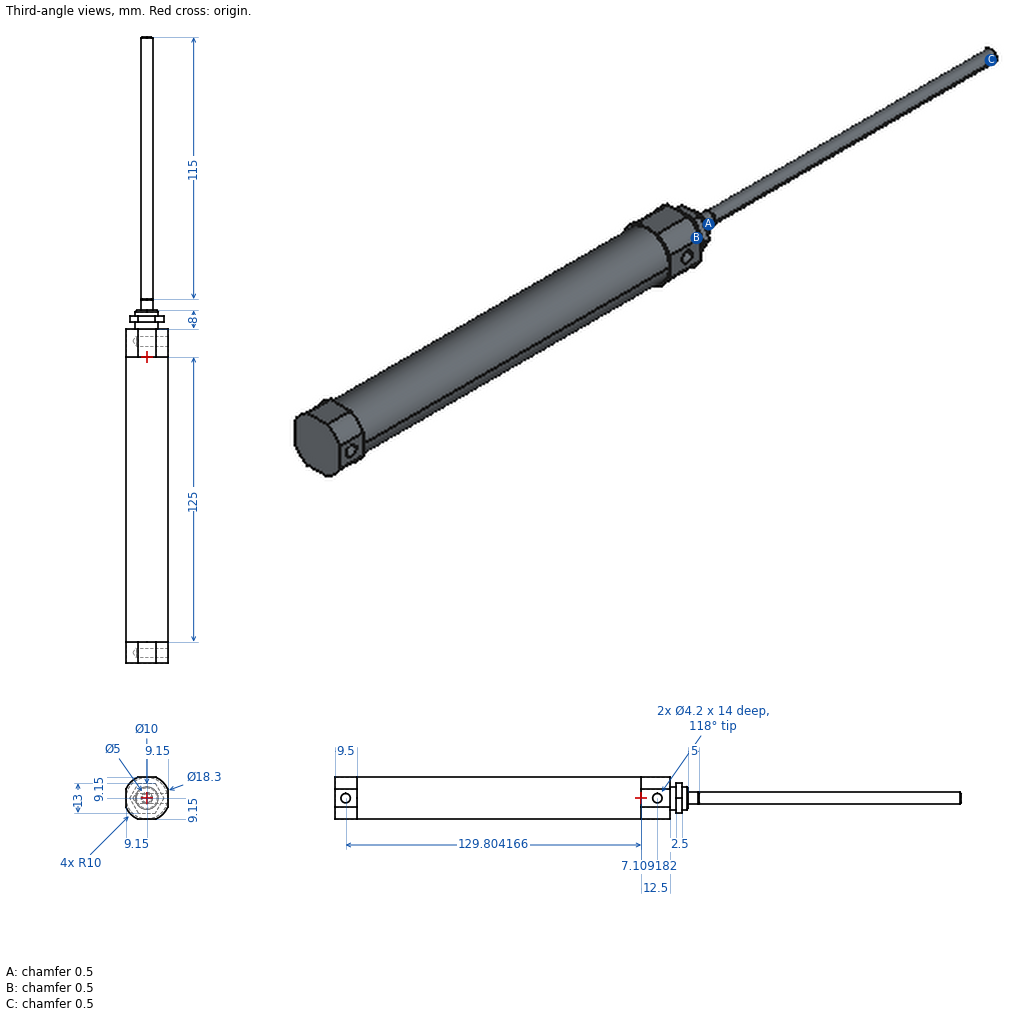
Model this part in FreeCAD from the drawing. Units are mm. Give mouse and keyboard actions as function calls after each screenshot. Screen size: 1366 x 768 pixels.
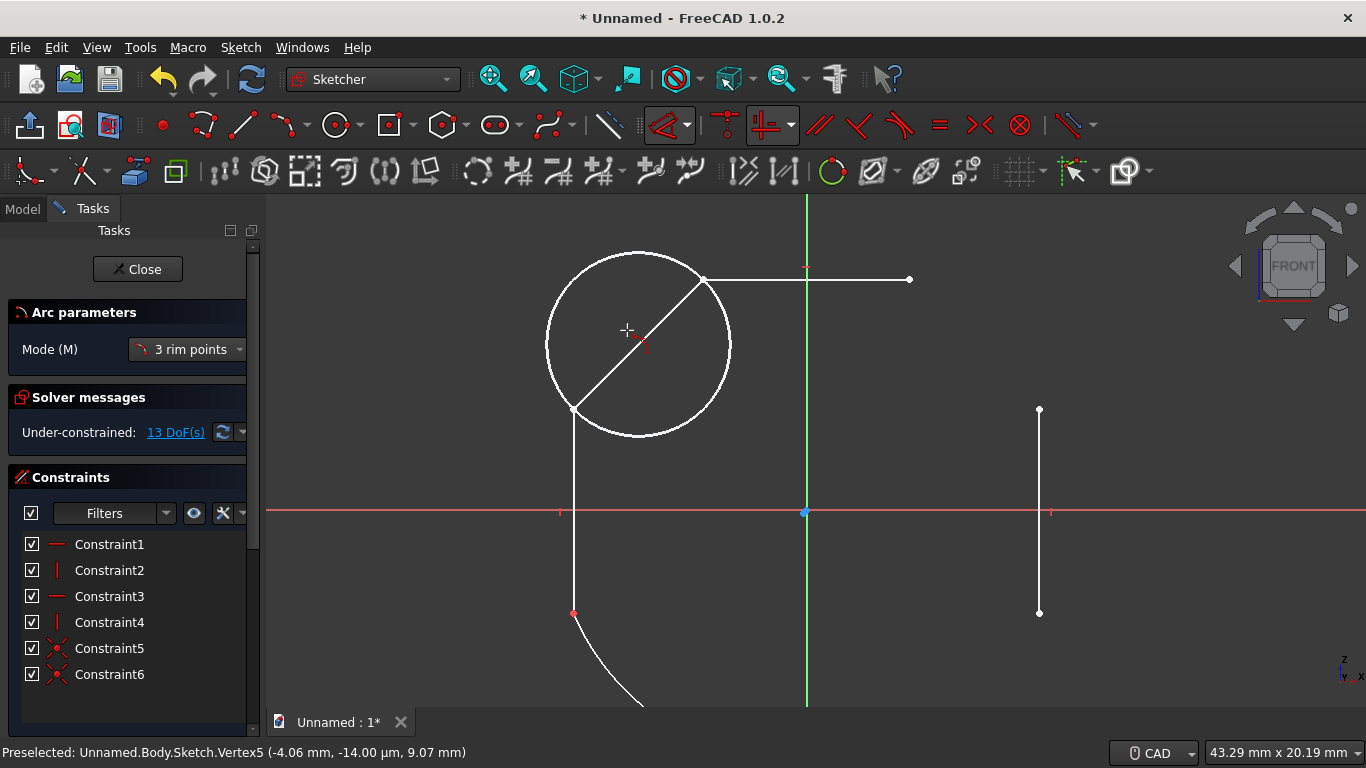
click(627, 330)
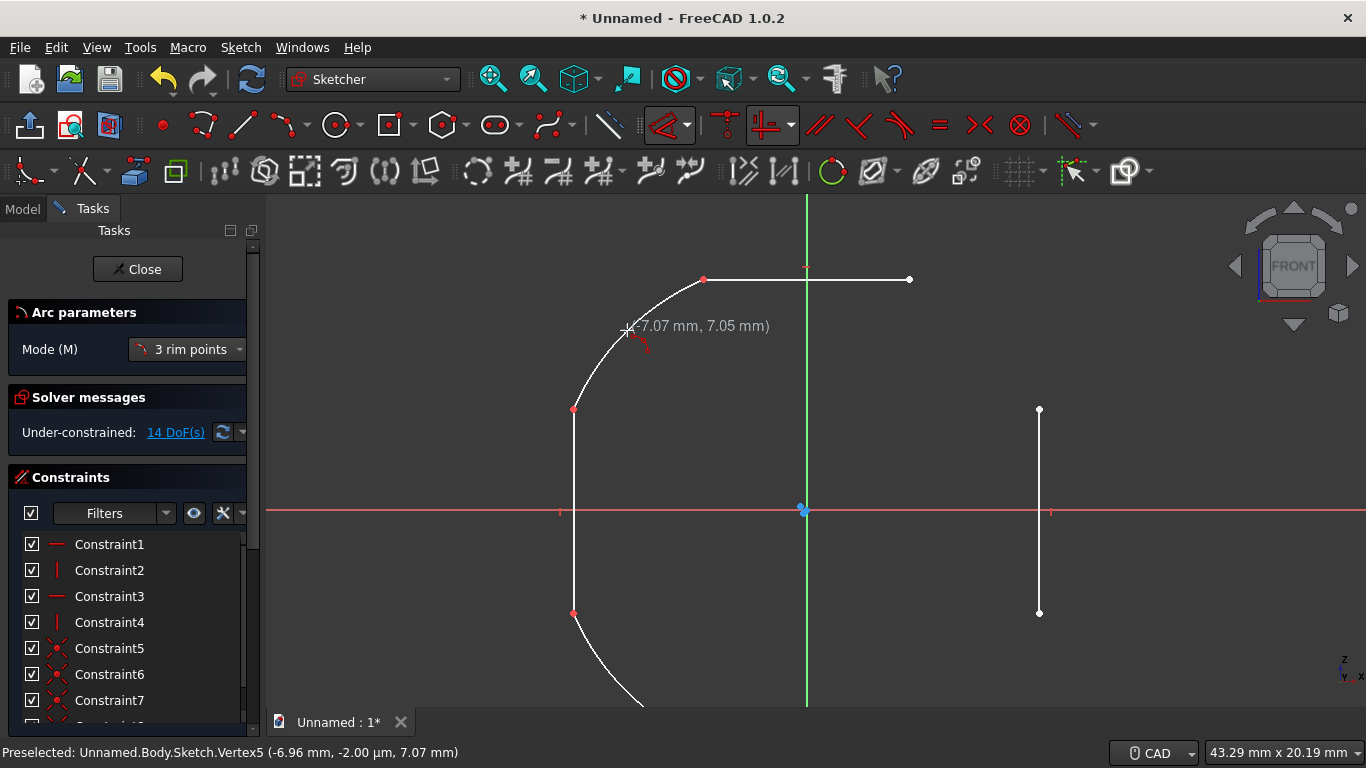
click(909, 280)
click(1039, 409)
click(986, 330)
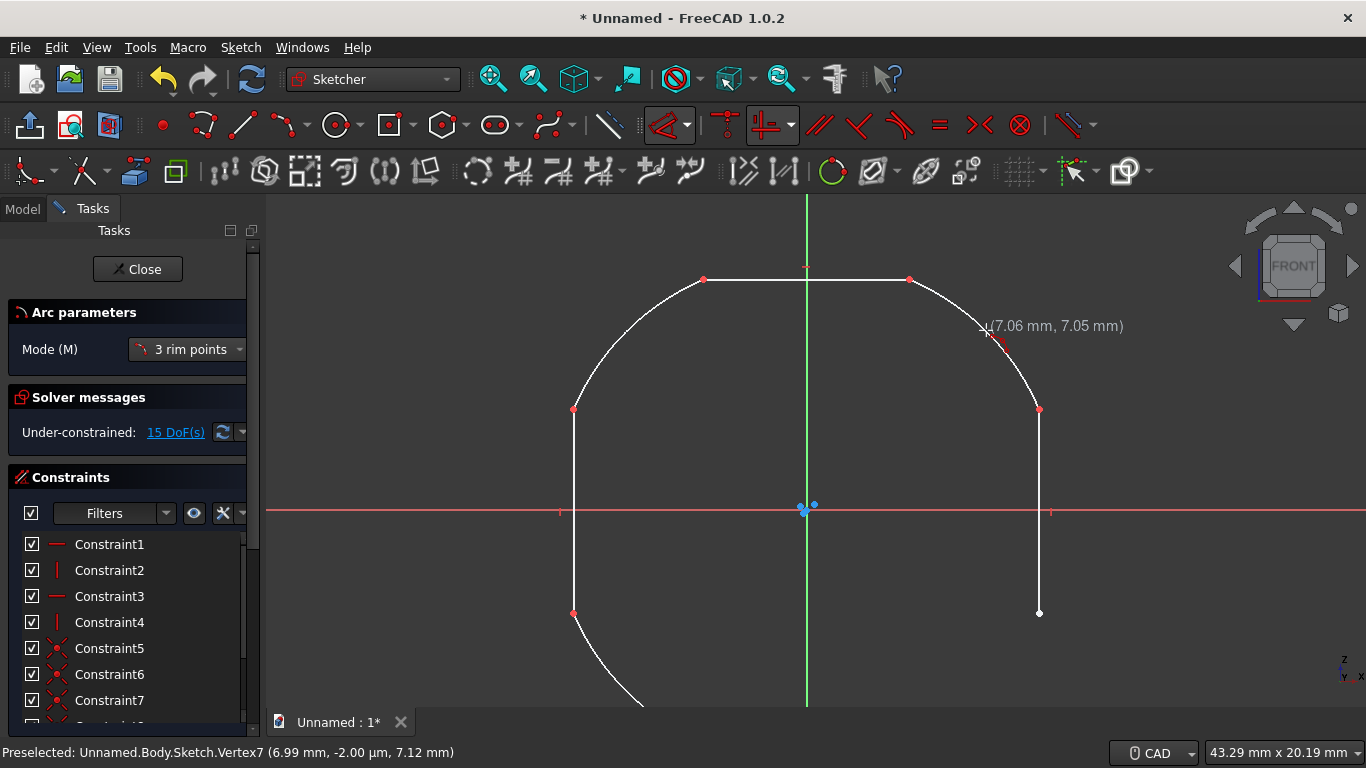
click(1039, 614)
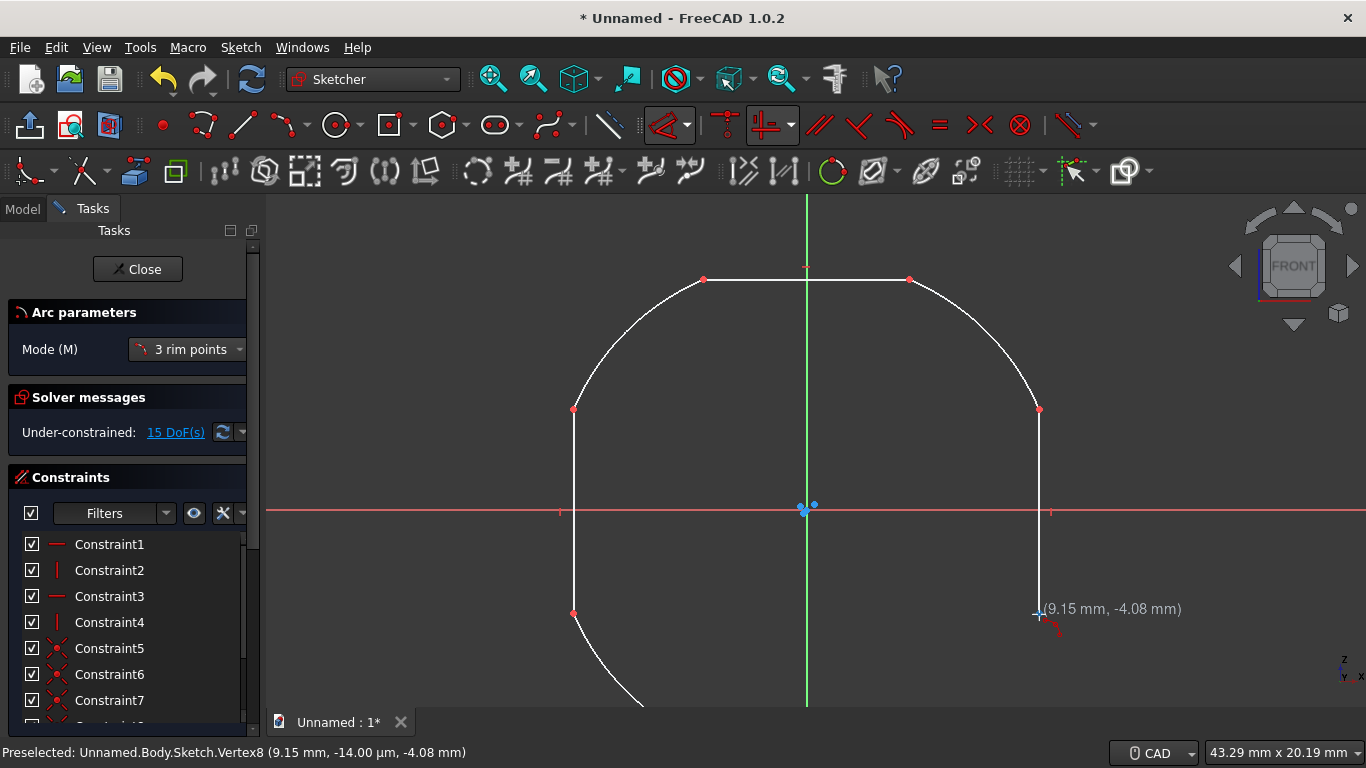
scroll(627, 329, down, 2)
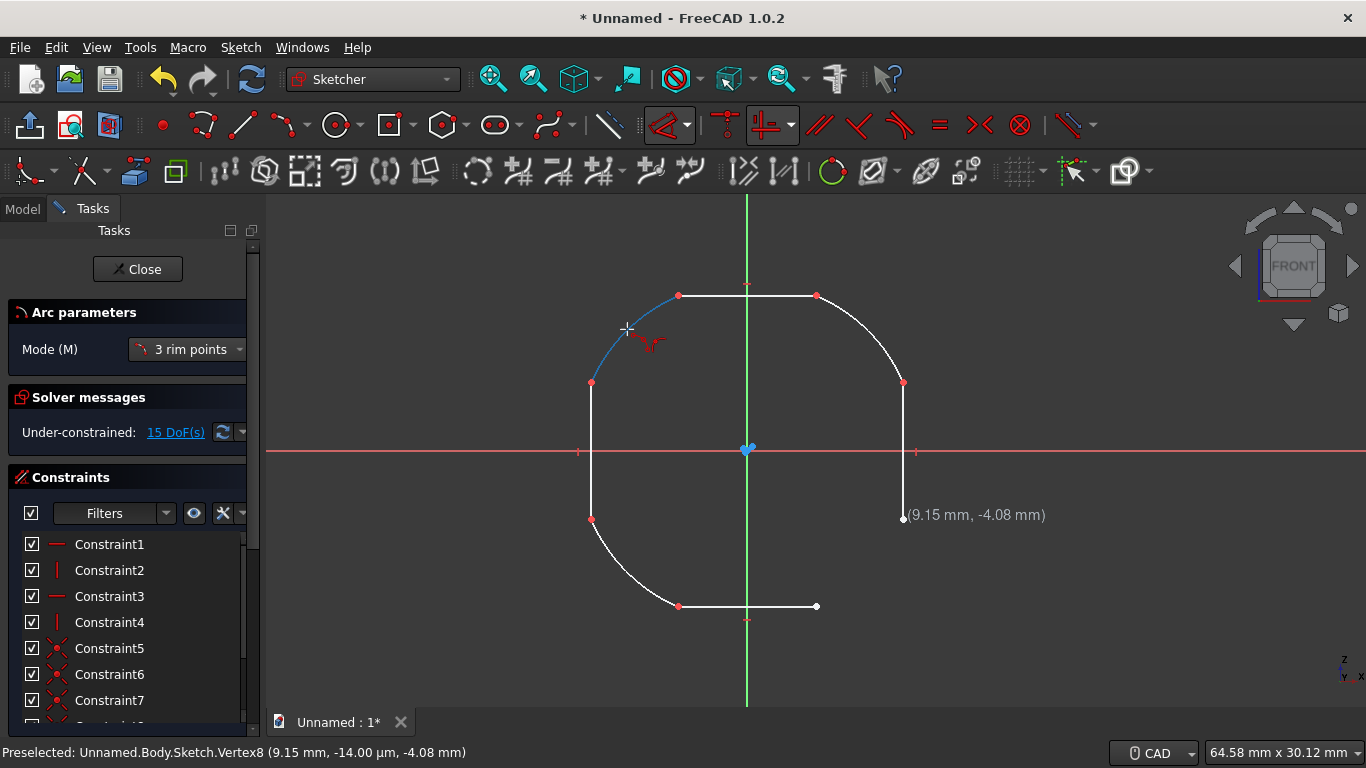
click(816, 607)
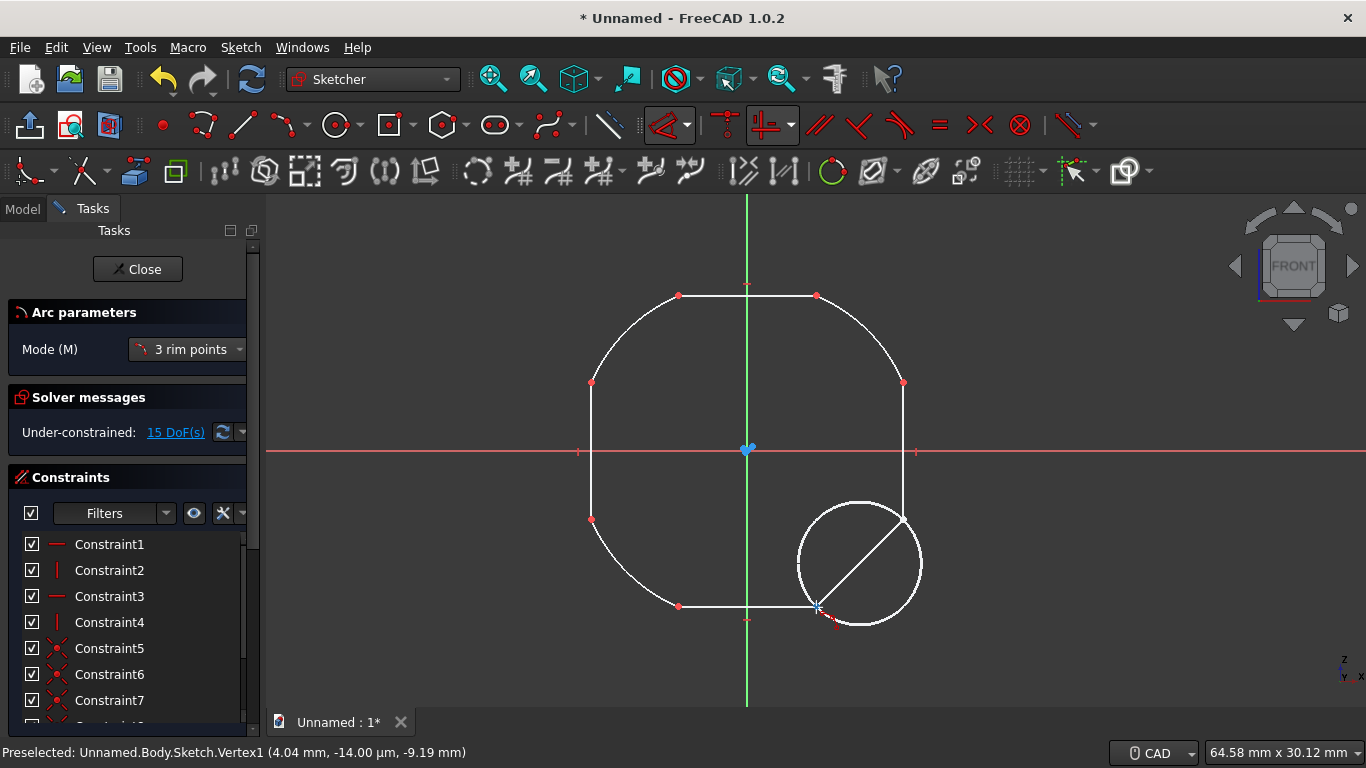
scroll(868, 571, up, 2)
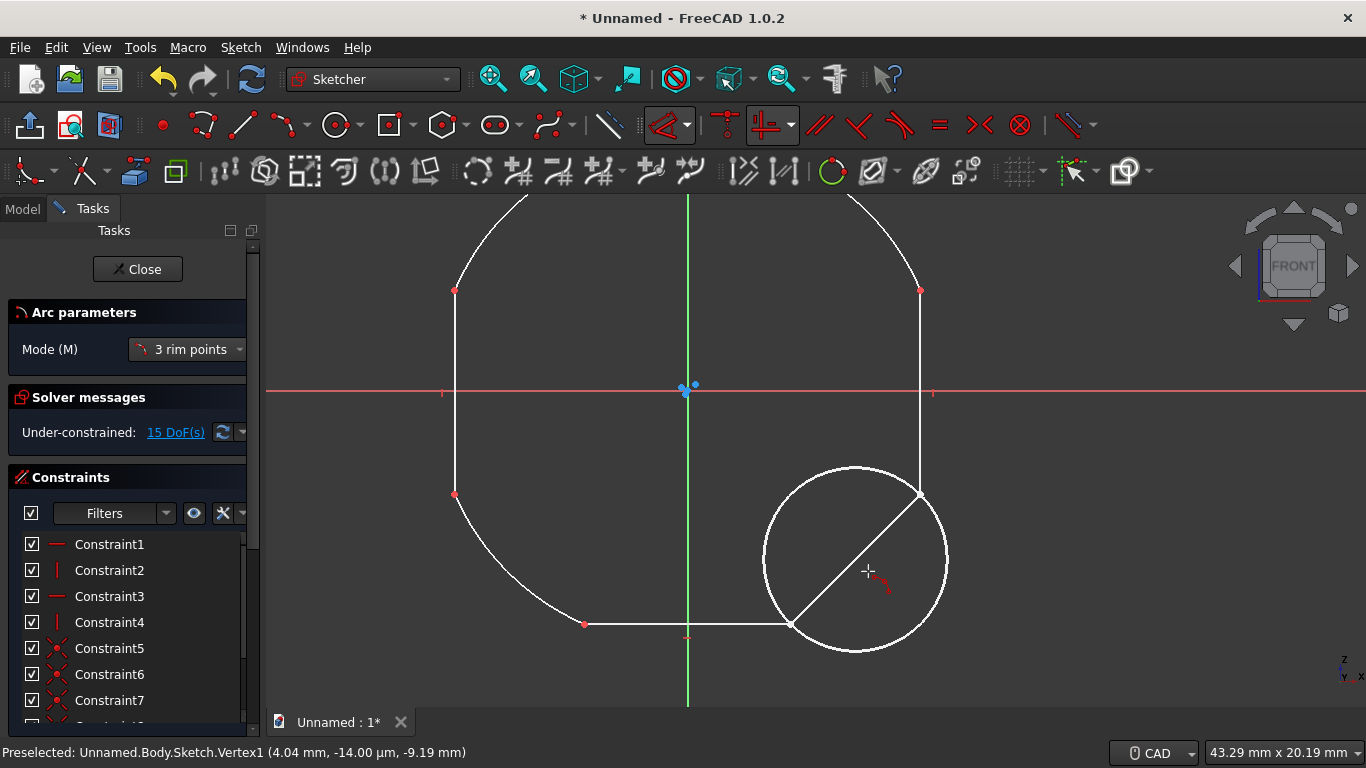
click(868, 571)
key(Escape)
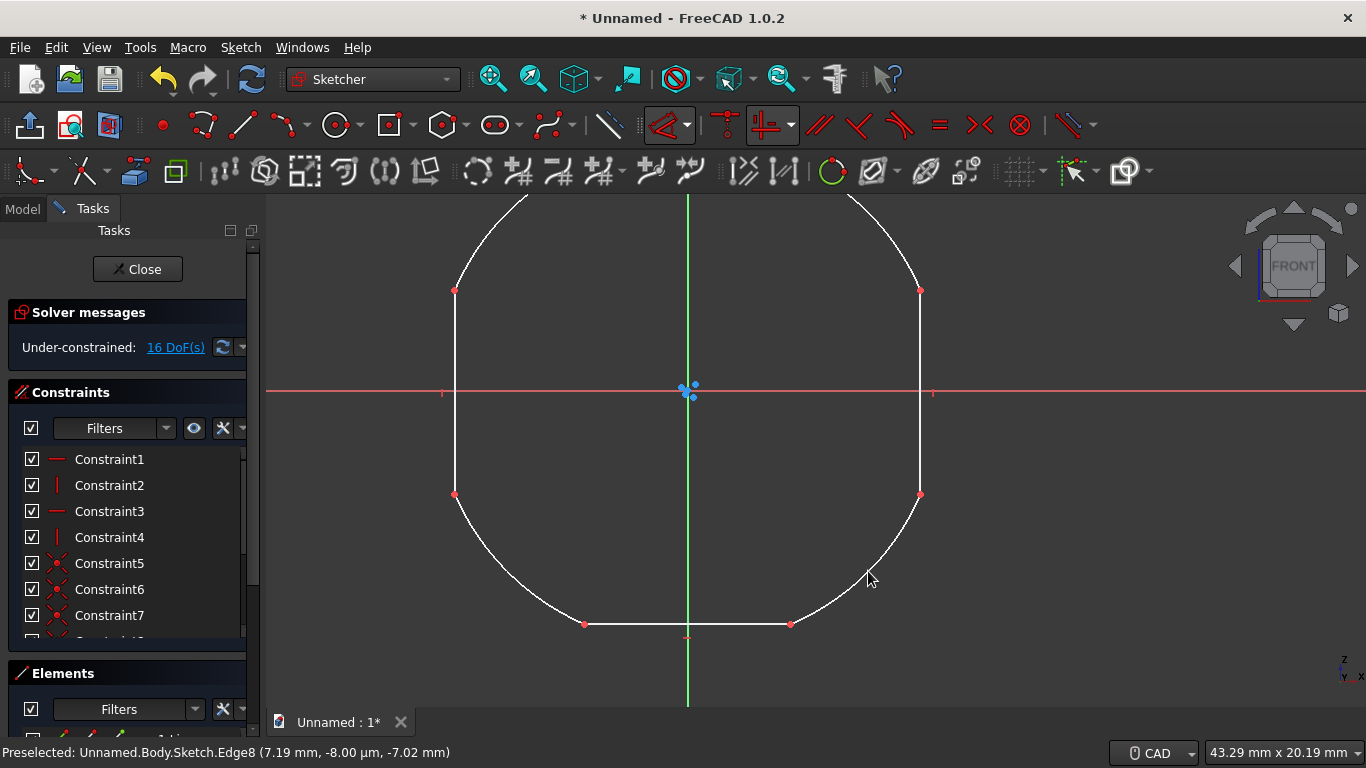
click(483, 543)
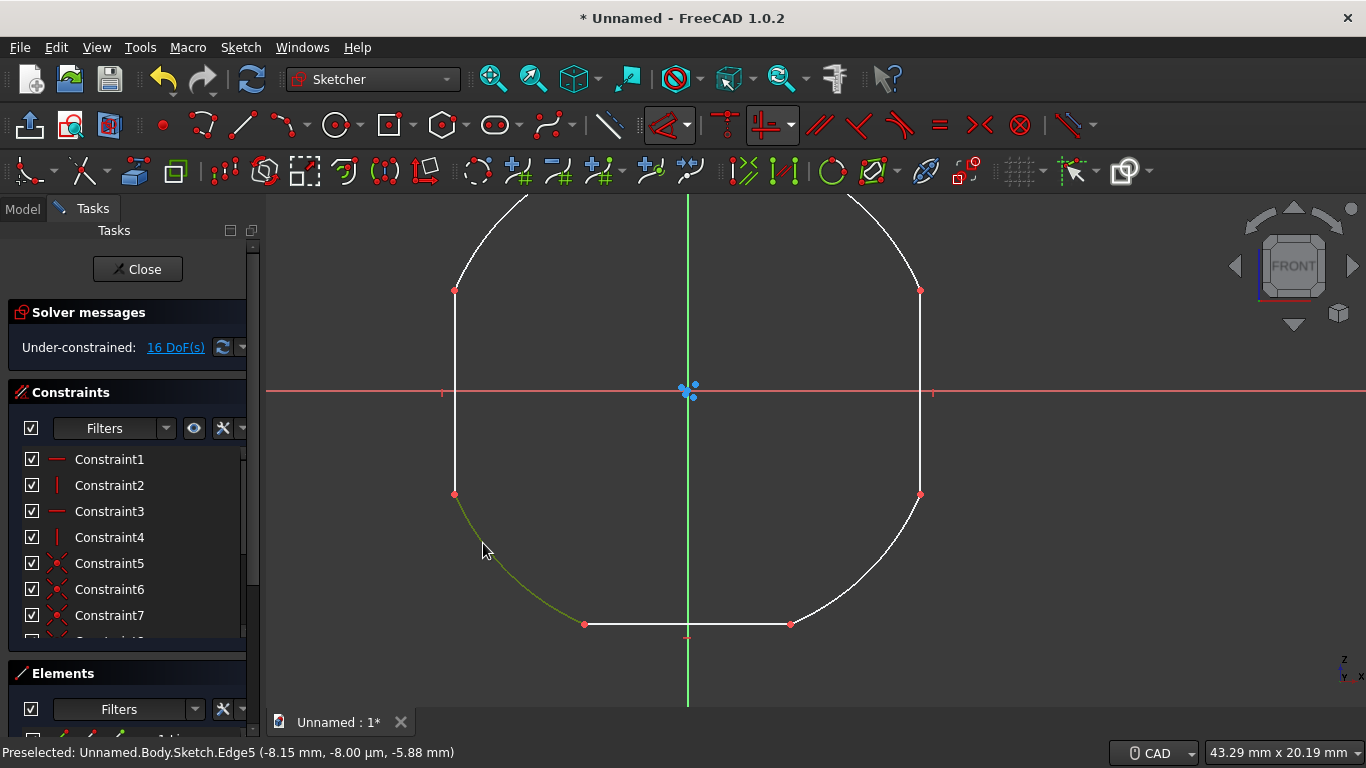
click(483, 241)